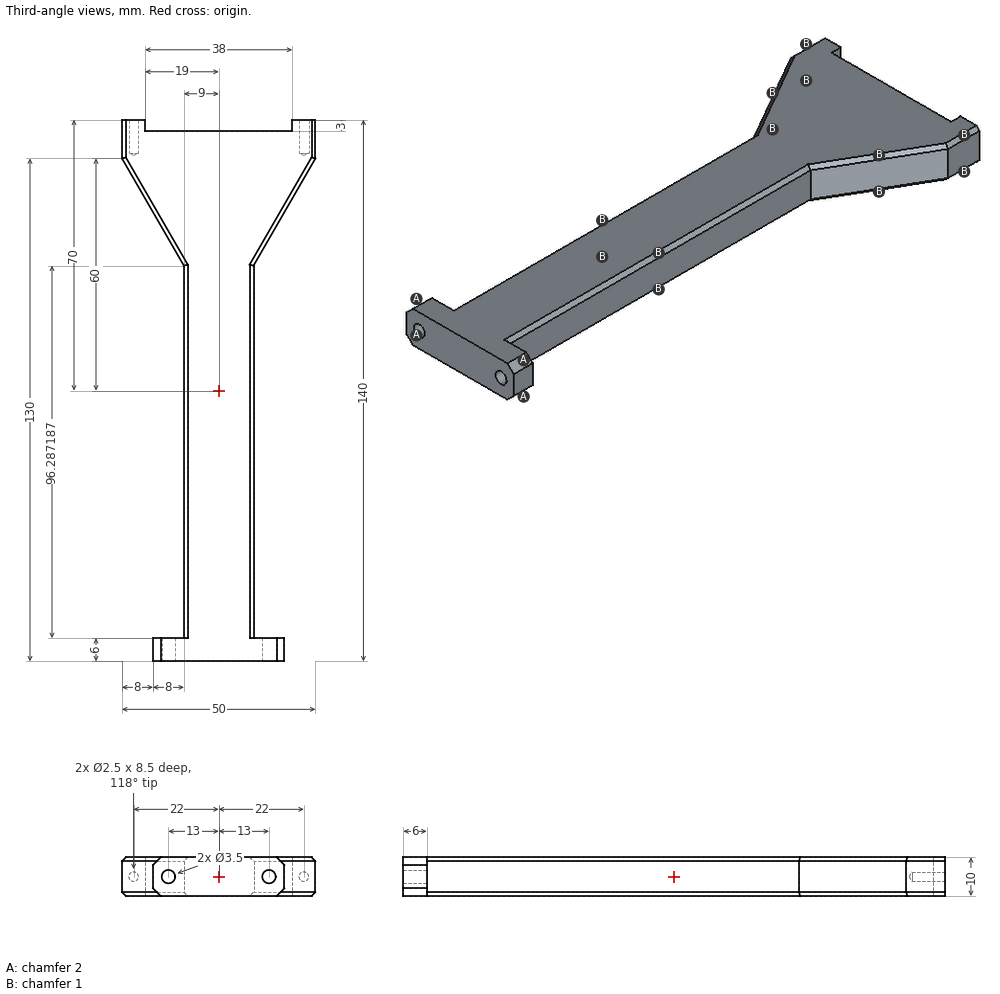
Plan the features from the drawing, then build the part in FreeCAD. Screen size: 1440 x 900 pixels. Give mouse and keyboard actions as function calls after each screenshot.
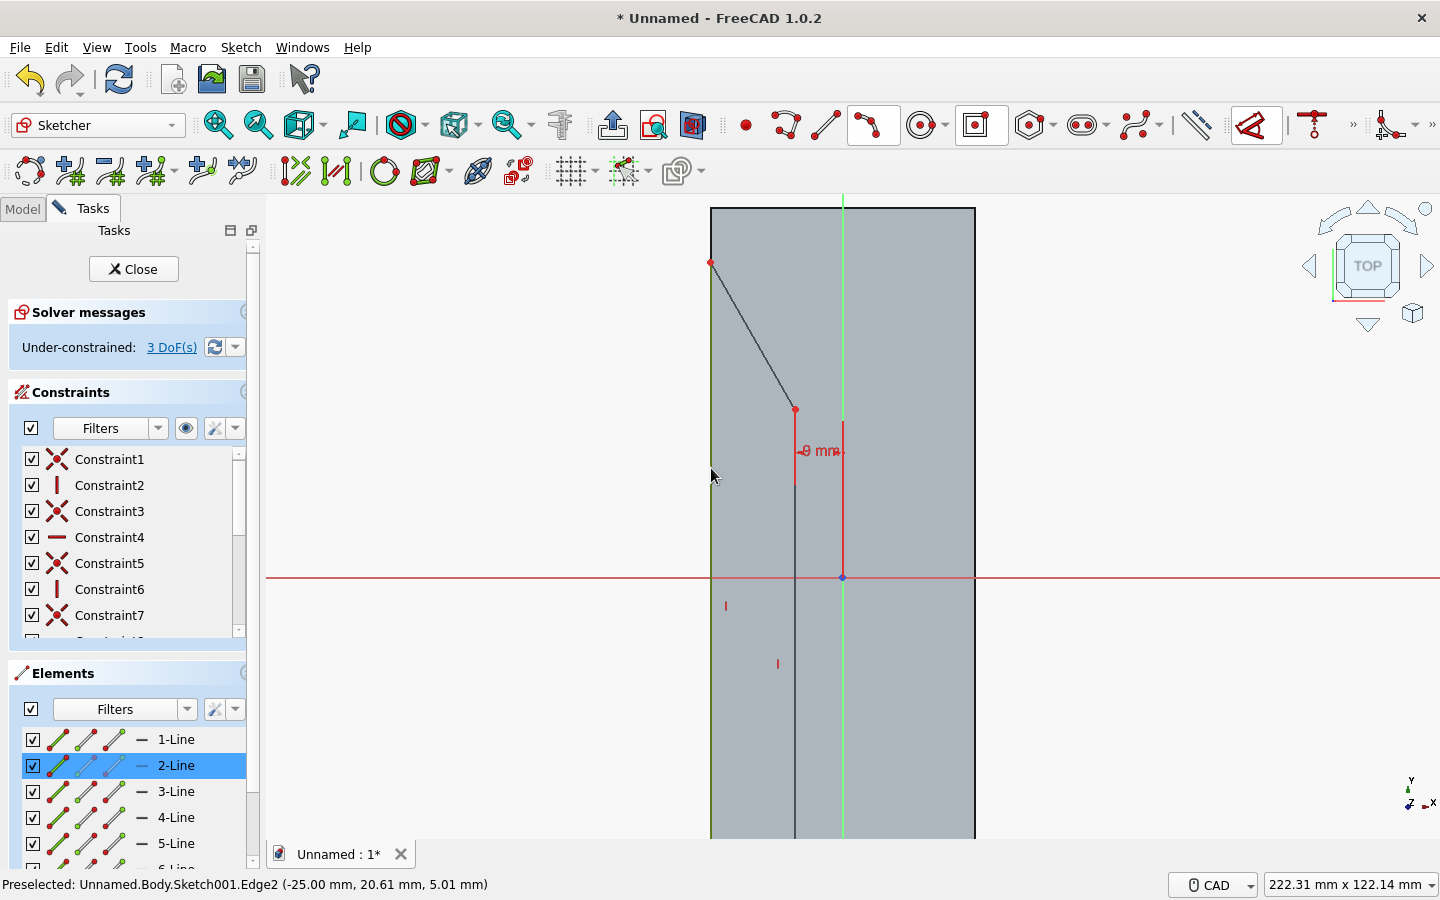
click(1276, 126)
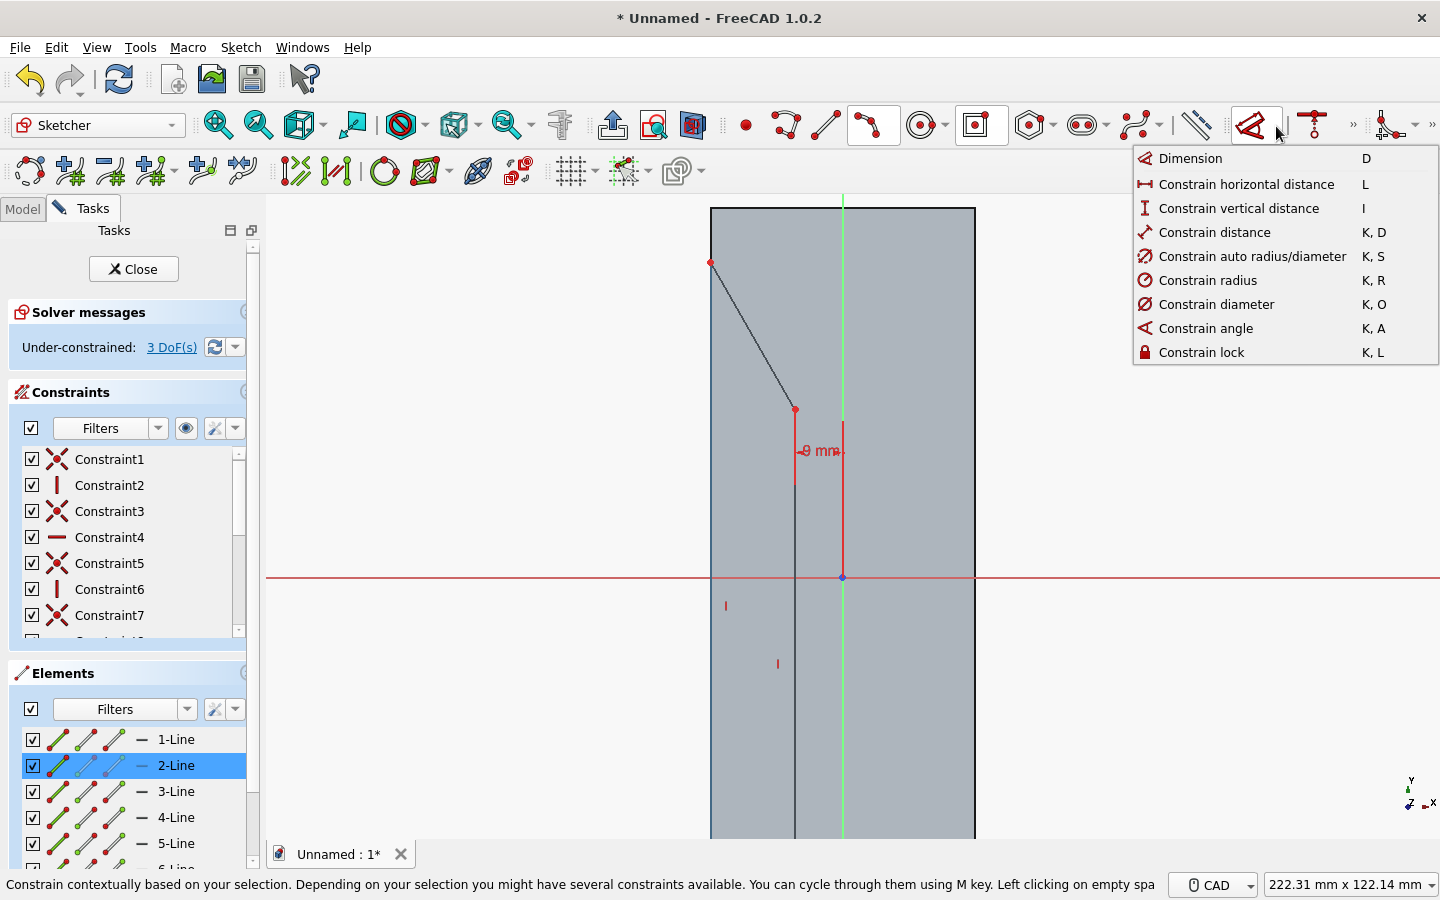
click(1286, 208)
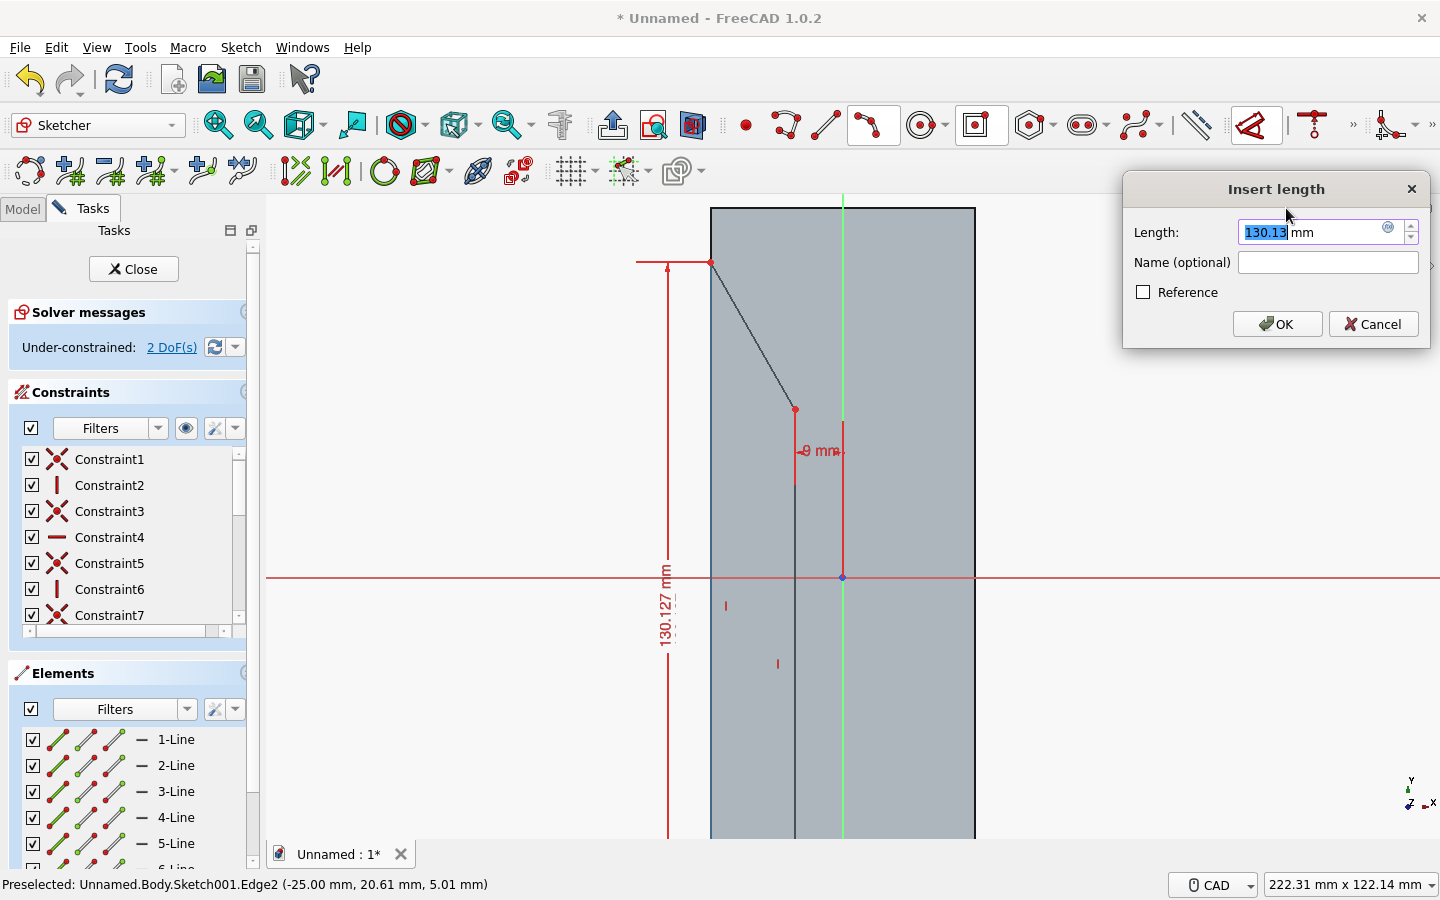
text(130)
key(Return)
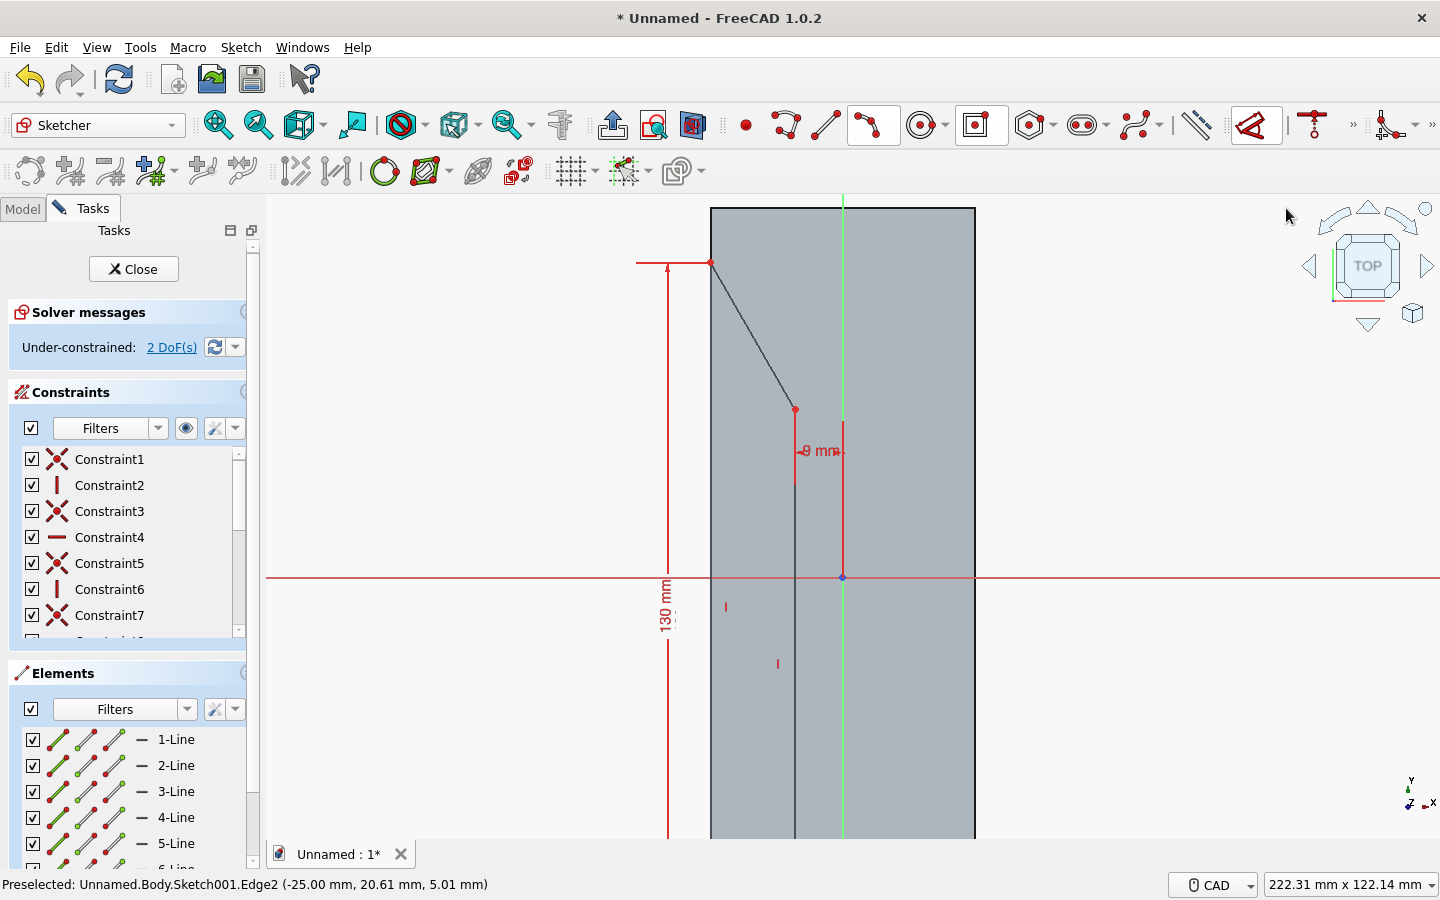
click(711, 263)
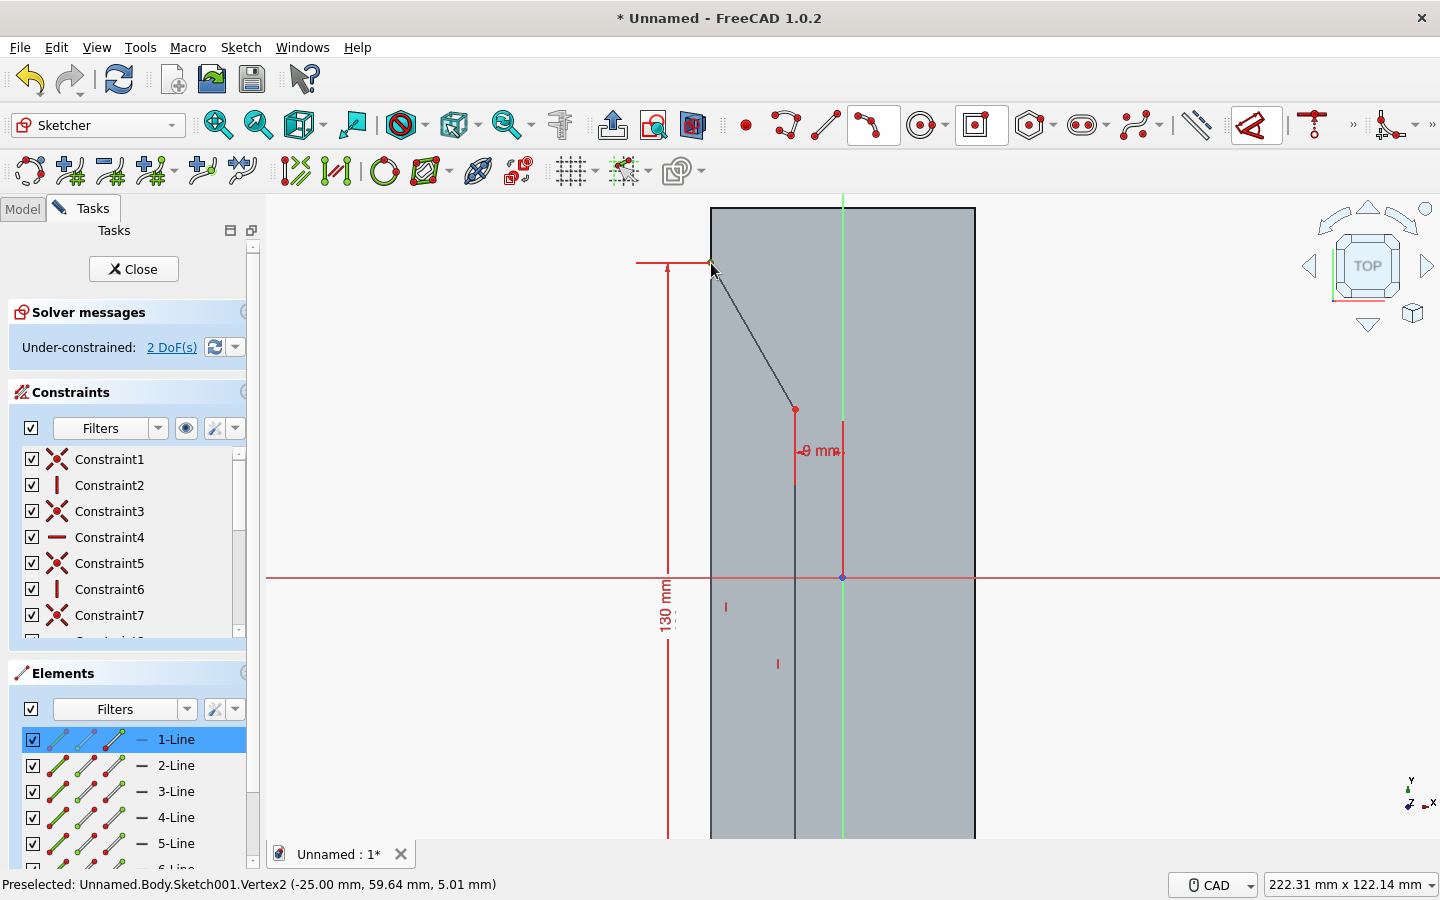
click(1276, 126)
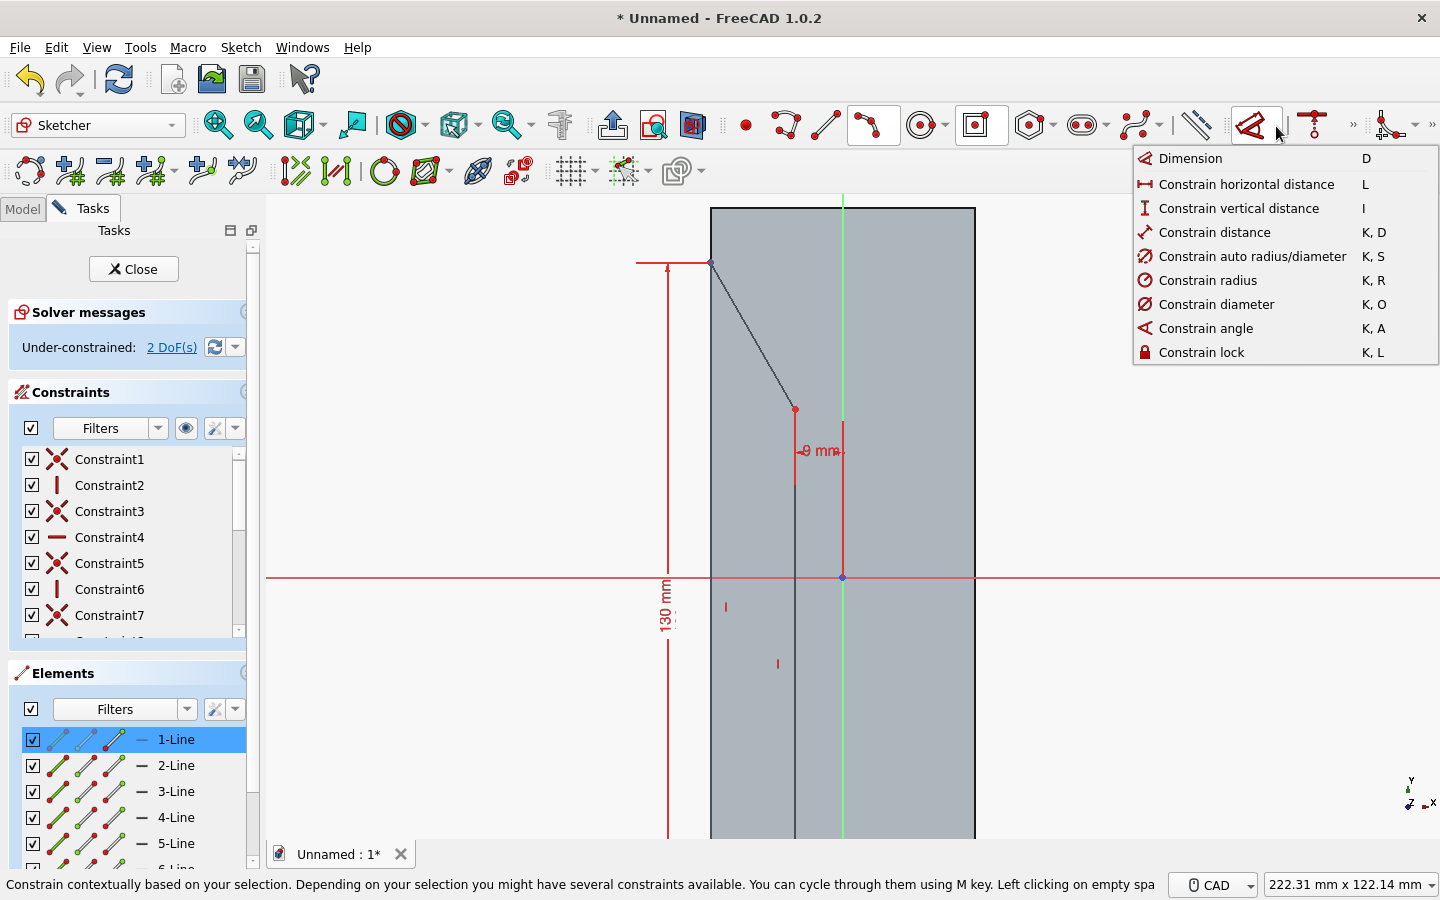
click(1286, 208)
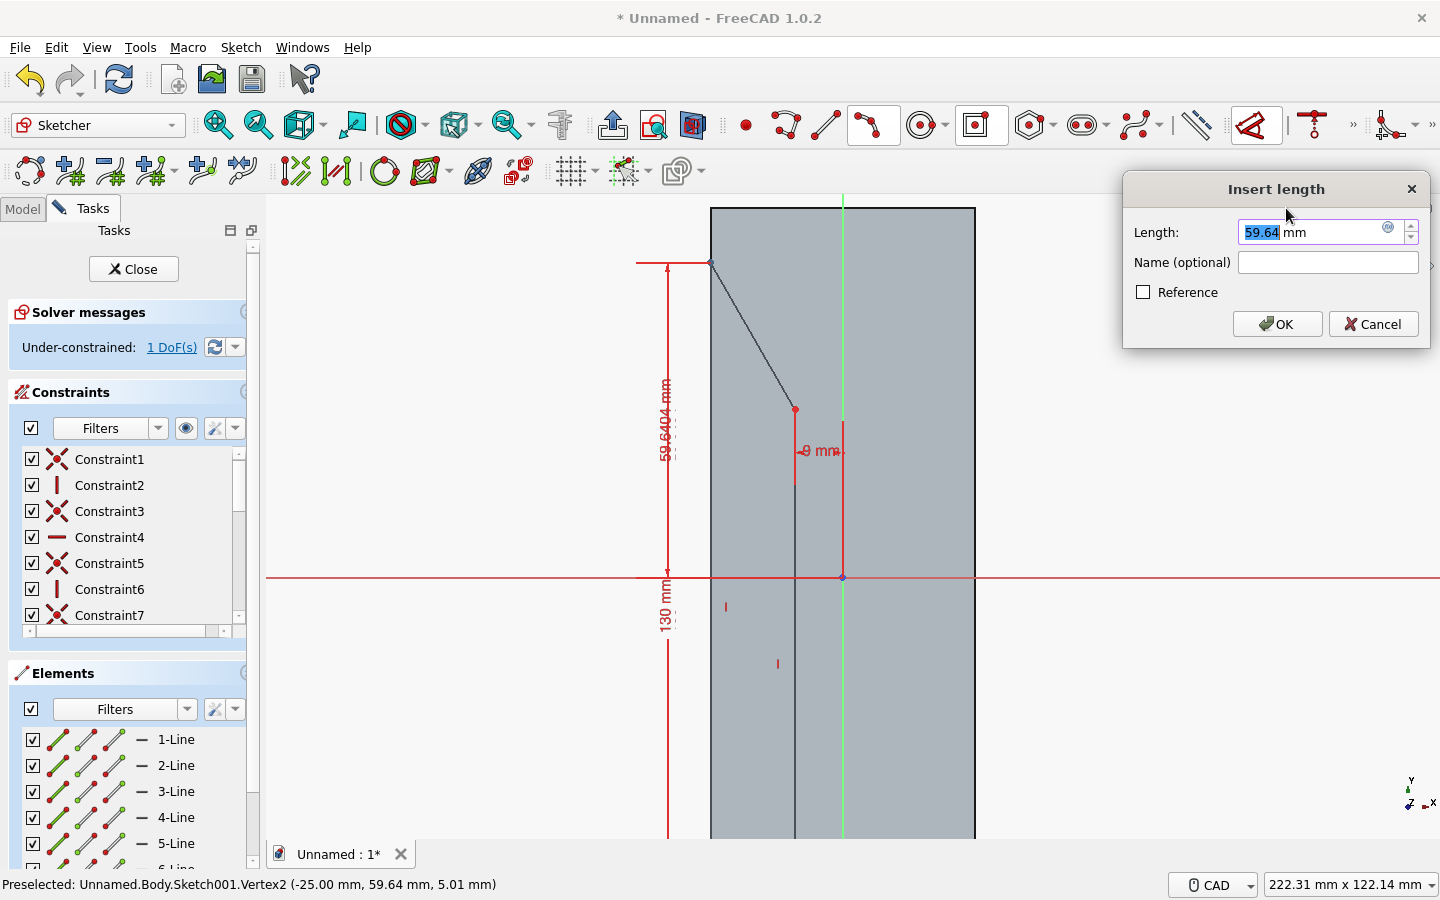
text(60)
key(Return)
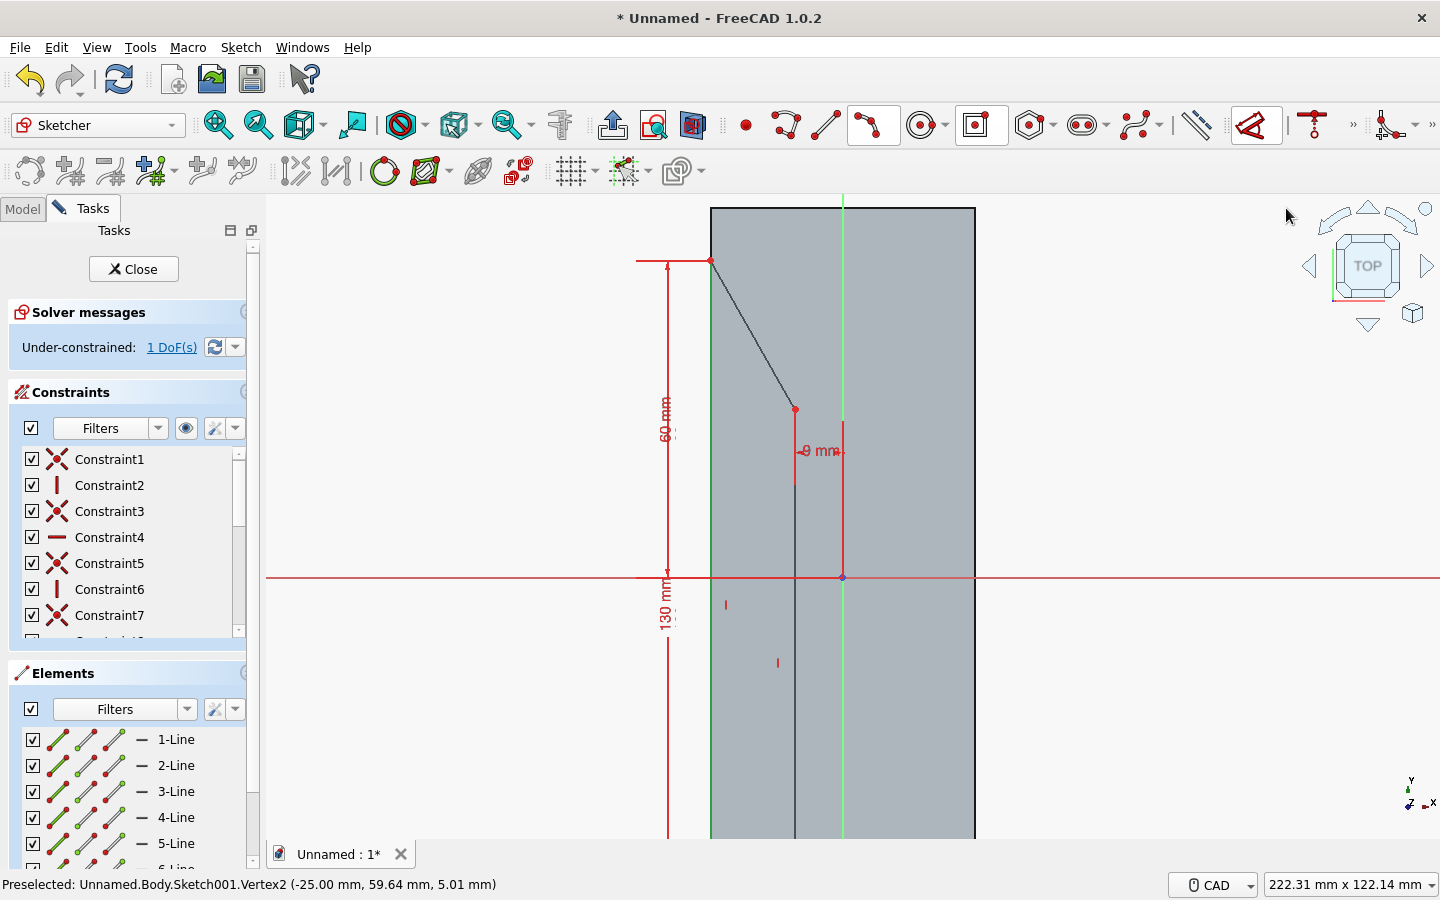
click(795, 764)